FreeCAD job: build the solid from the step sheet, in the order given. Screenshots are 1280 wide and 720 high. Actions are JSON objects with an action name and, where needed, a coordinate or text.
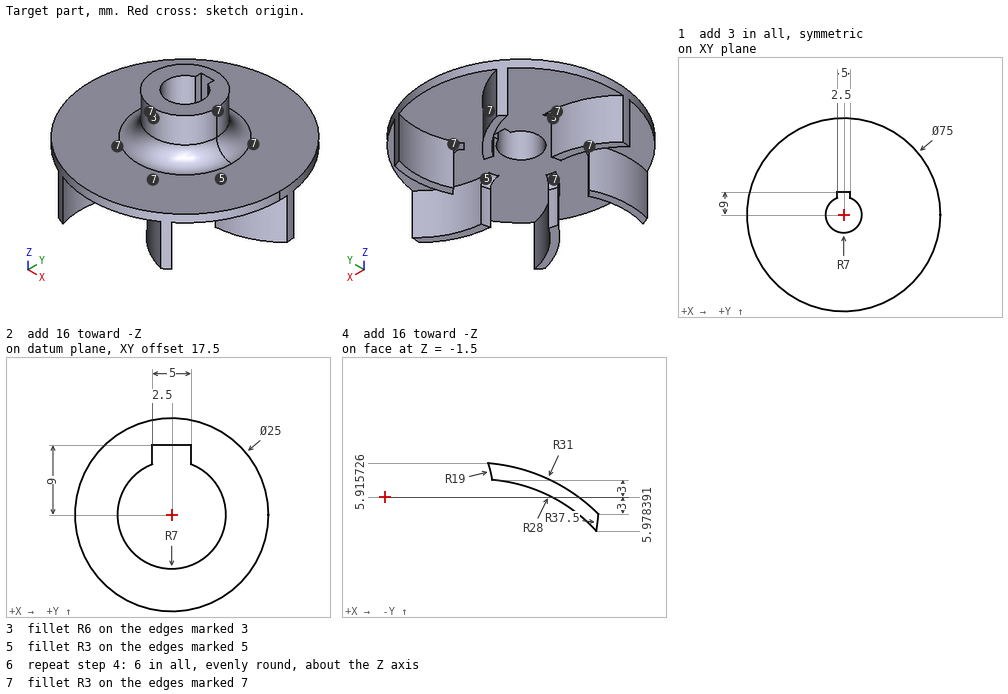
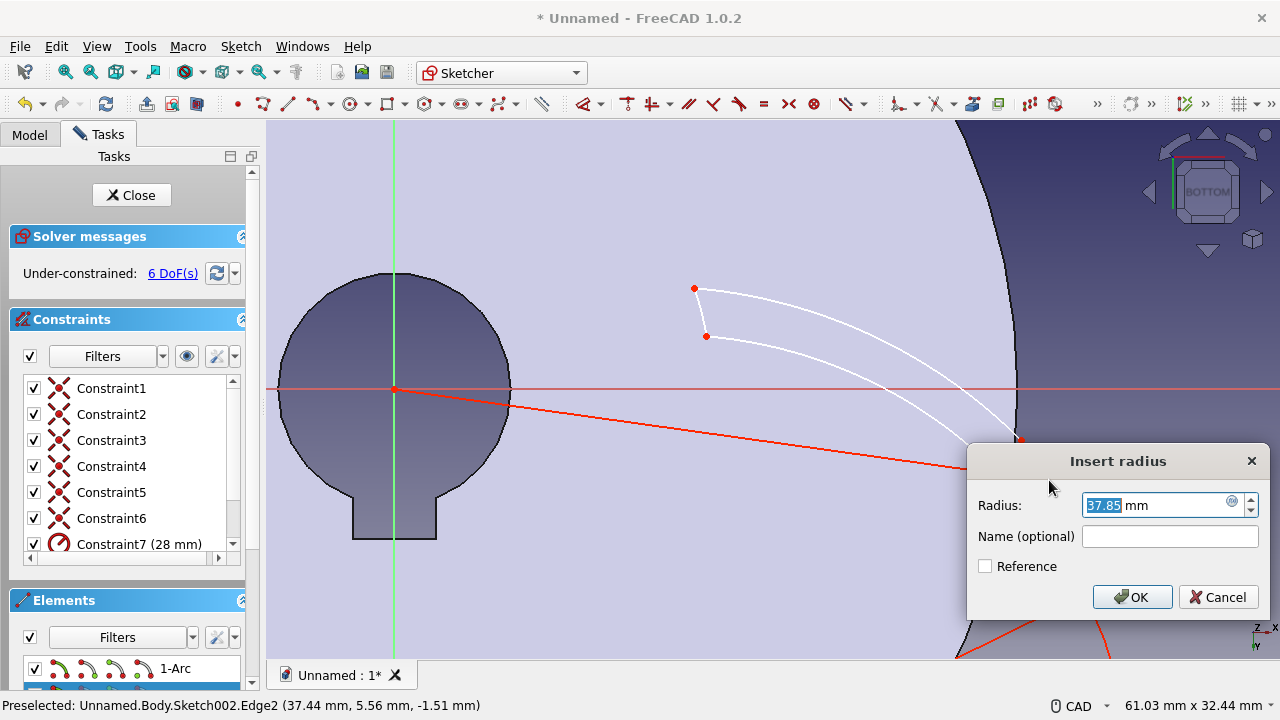
{"action": "type", "text": "37.5"}
{"action": "key", "text": "Return"}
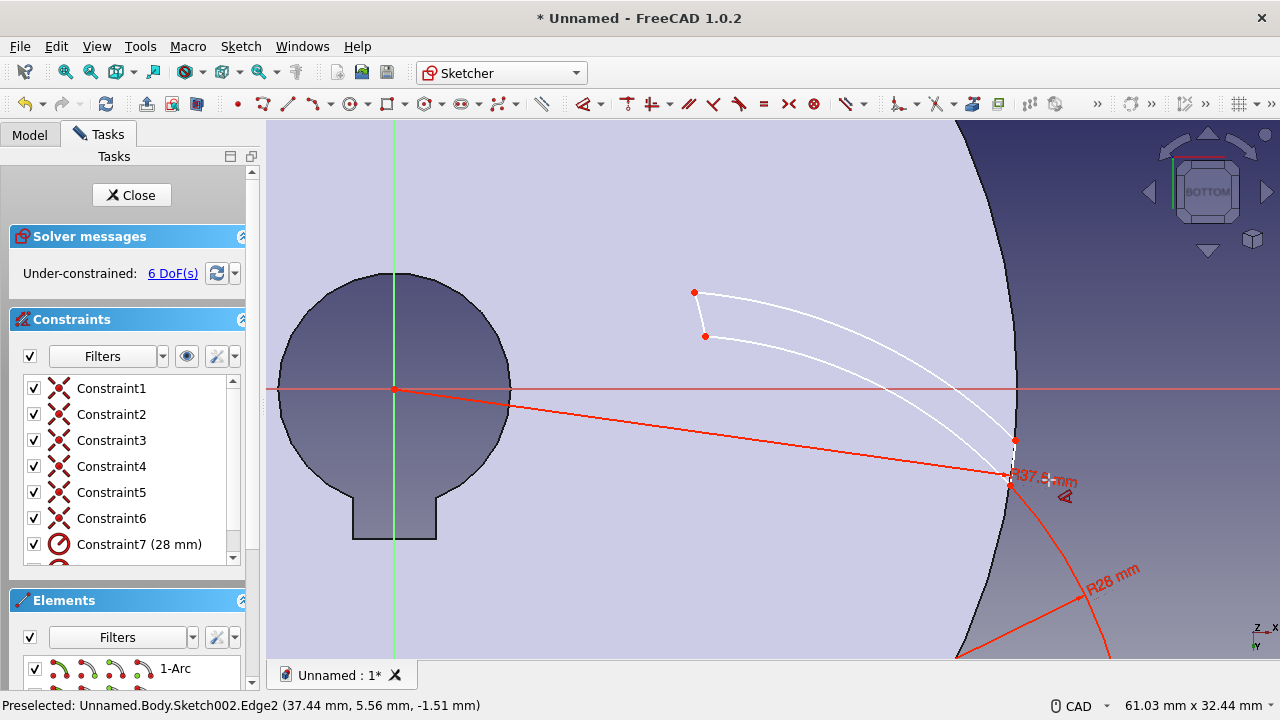
{"action": "left_click", "coordinate": [931, 373]}
{"action": "left_click", "coordinate": [948, 346]}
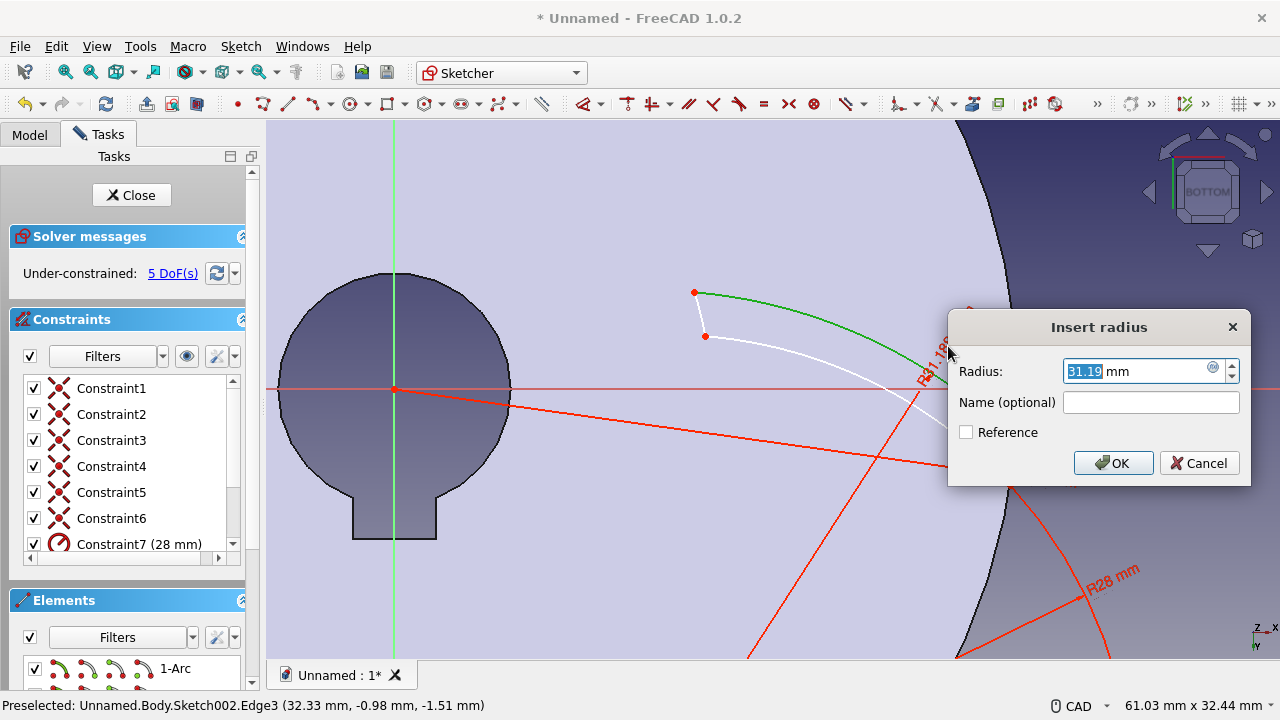
{"action": "type", "text": "31"}
{"action": "key", "text": "Return"}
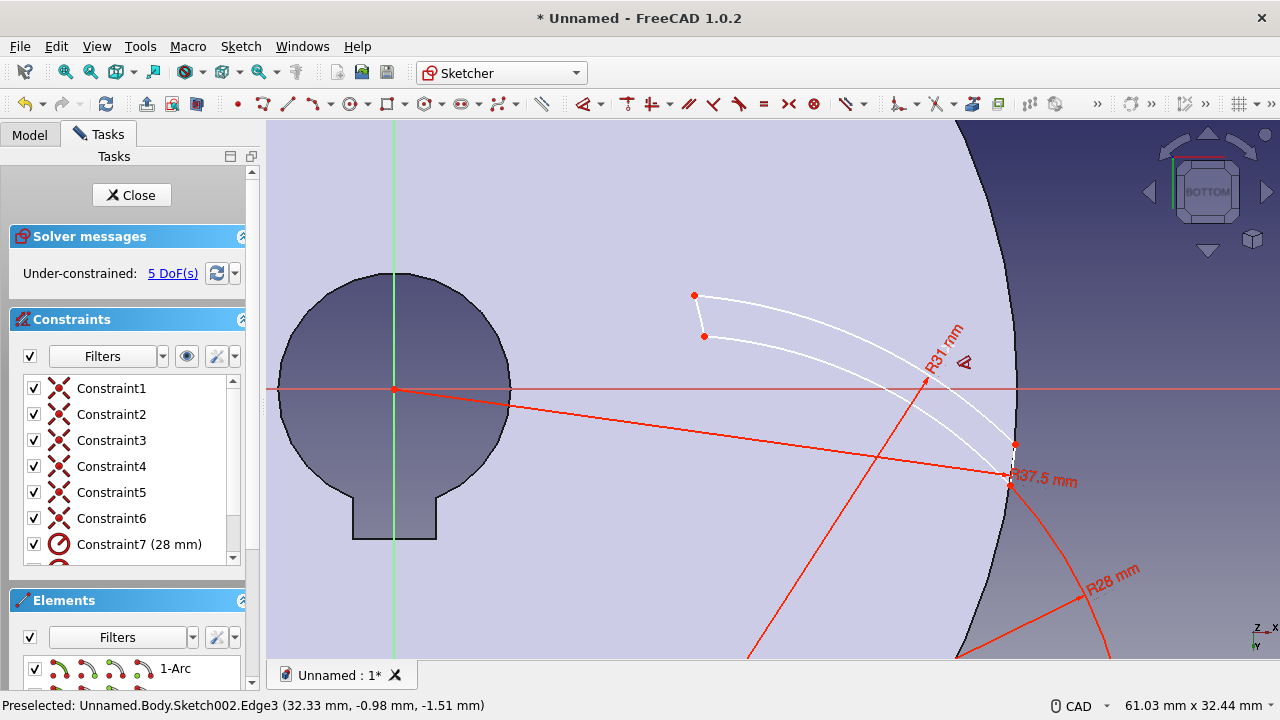
{"action": "left_click", "coordinate": [702, 324]}
{"action": "left_click", "coordinate": [733, 317]}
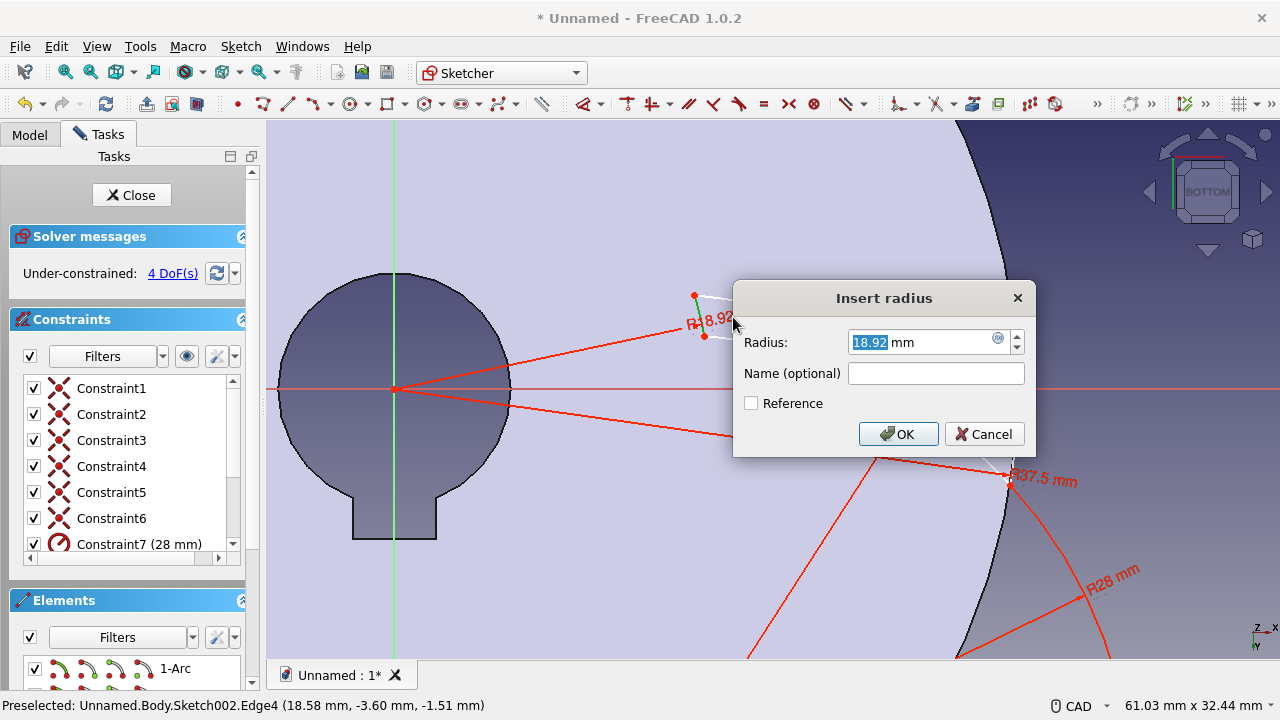
{"action": "type", "text": "19"}
{"action": "key", "text": "Return"}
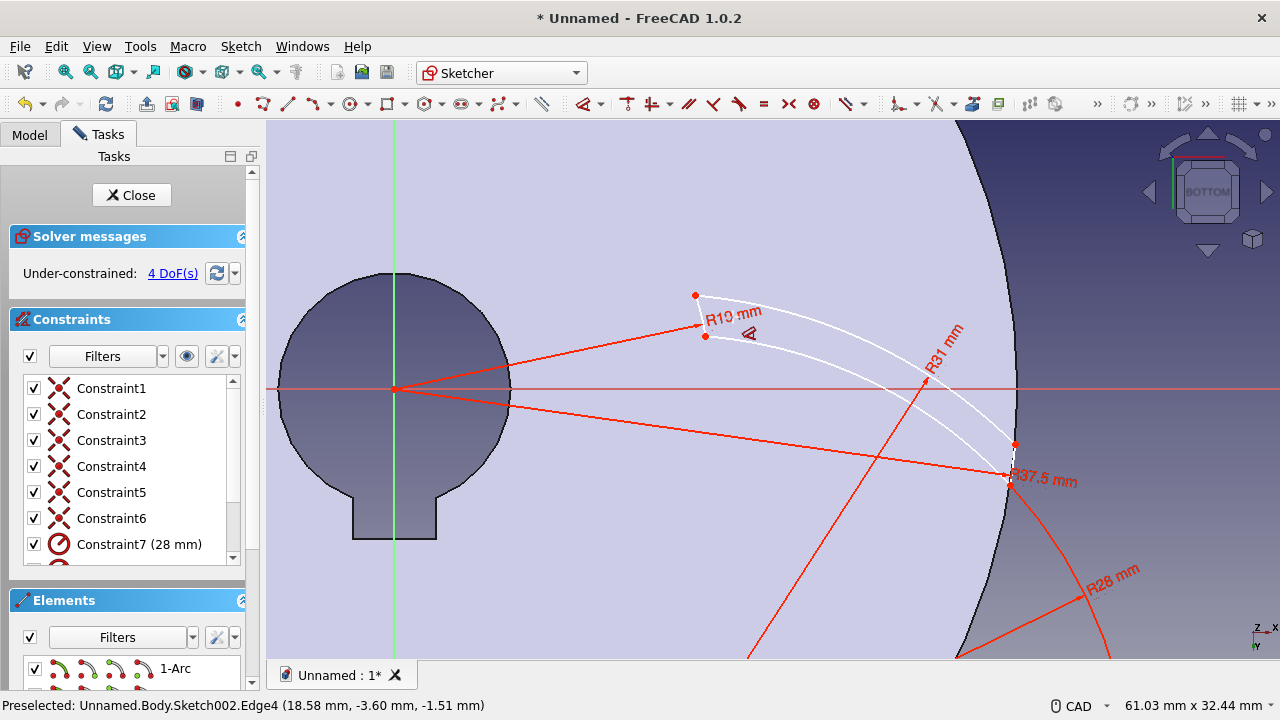
{"action": "left_click", "coordinate": [706, 336]}
{"action": "left_click", "coordinate": [360, 363]}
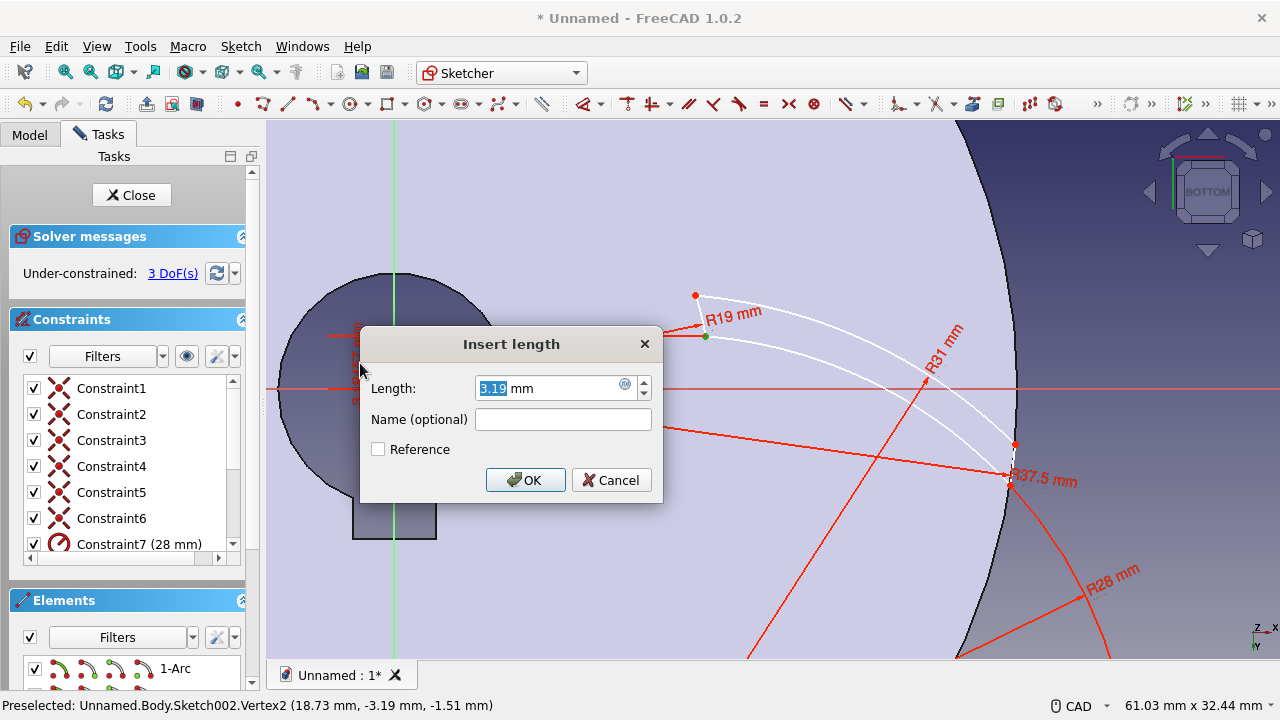
{"action": "type", "text": "3"}
{"action": "key", "text": "Return"}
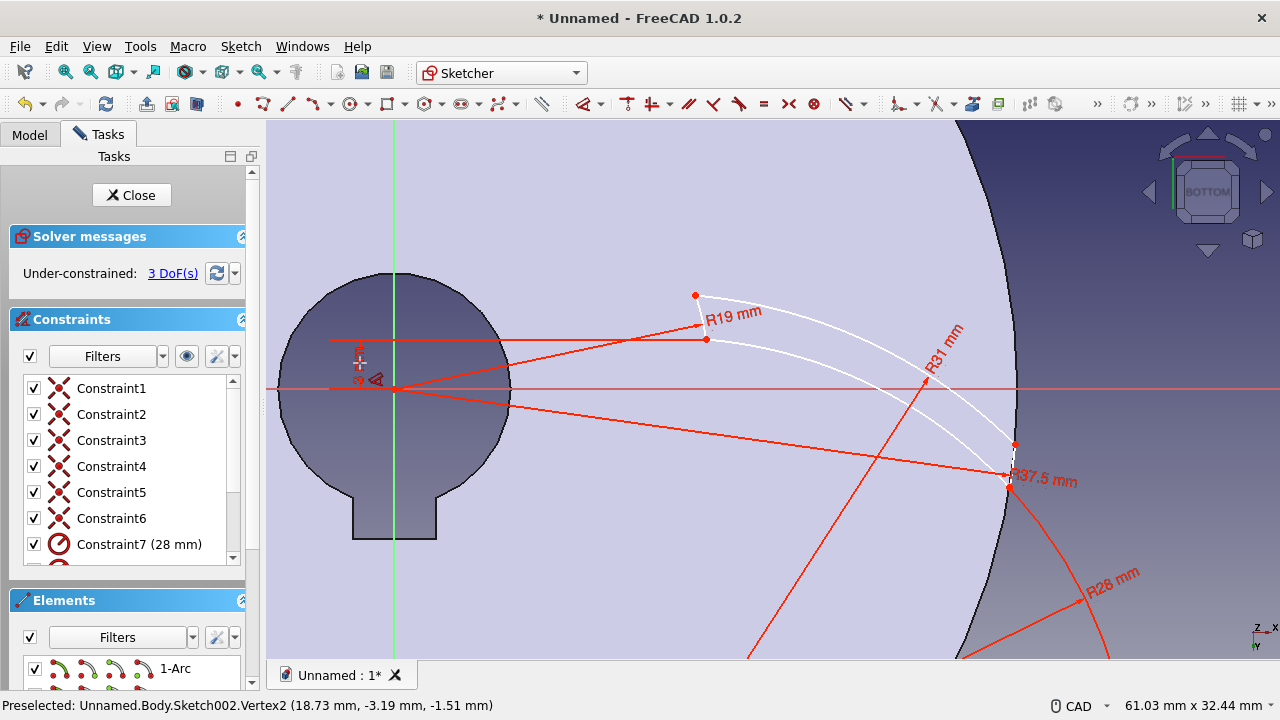
{"action": "left_click", "coordinate": [1015, 445]}
{"action": "left_click", "coordinate": [360, 417]}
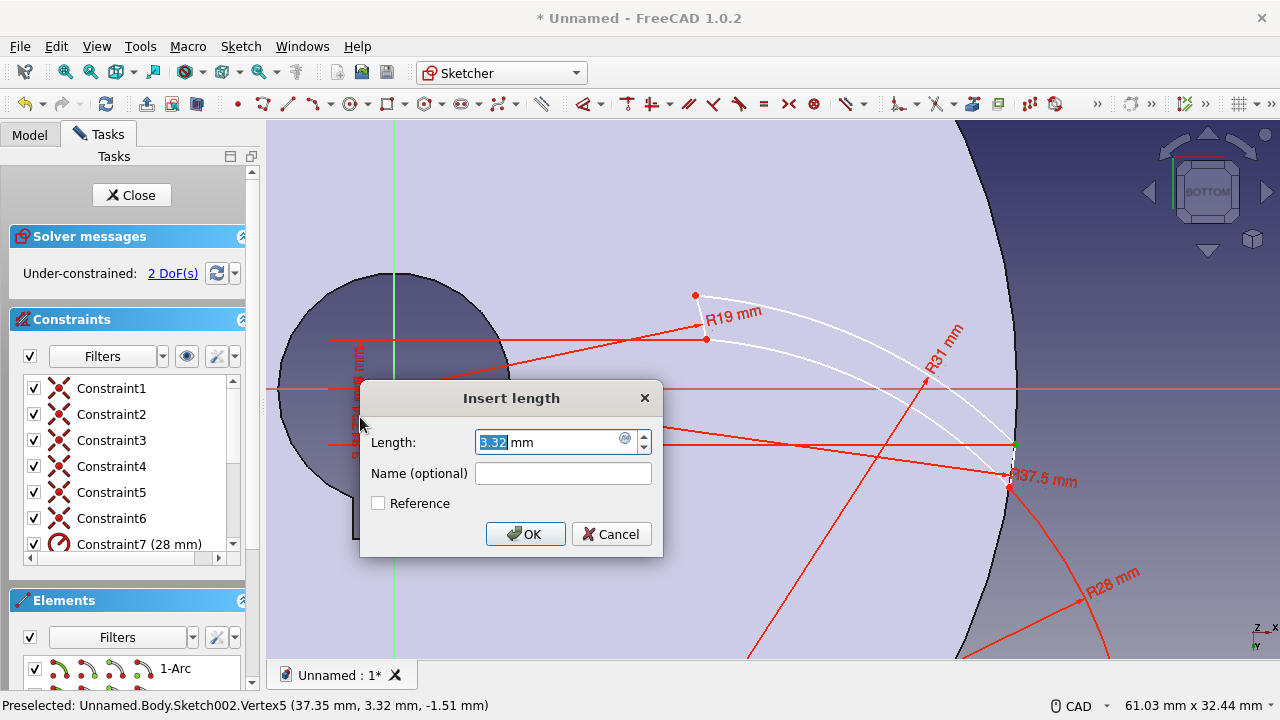
{"action": "type", "text": "3"}
{"action": "key", "text": "Return"}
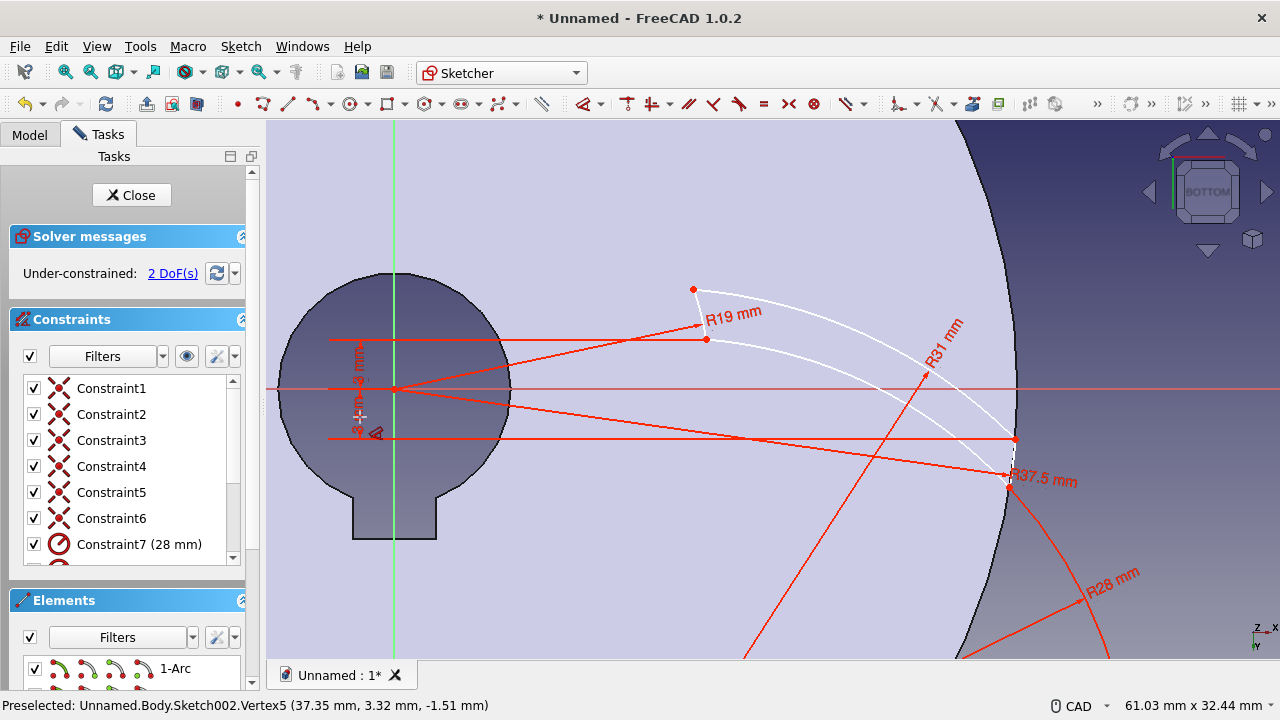
{"action": "left_click", "coordinate": [1010, 488]}
{"action": "left_click", "coordinate": [360, 439]}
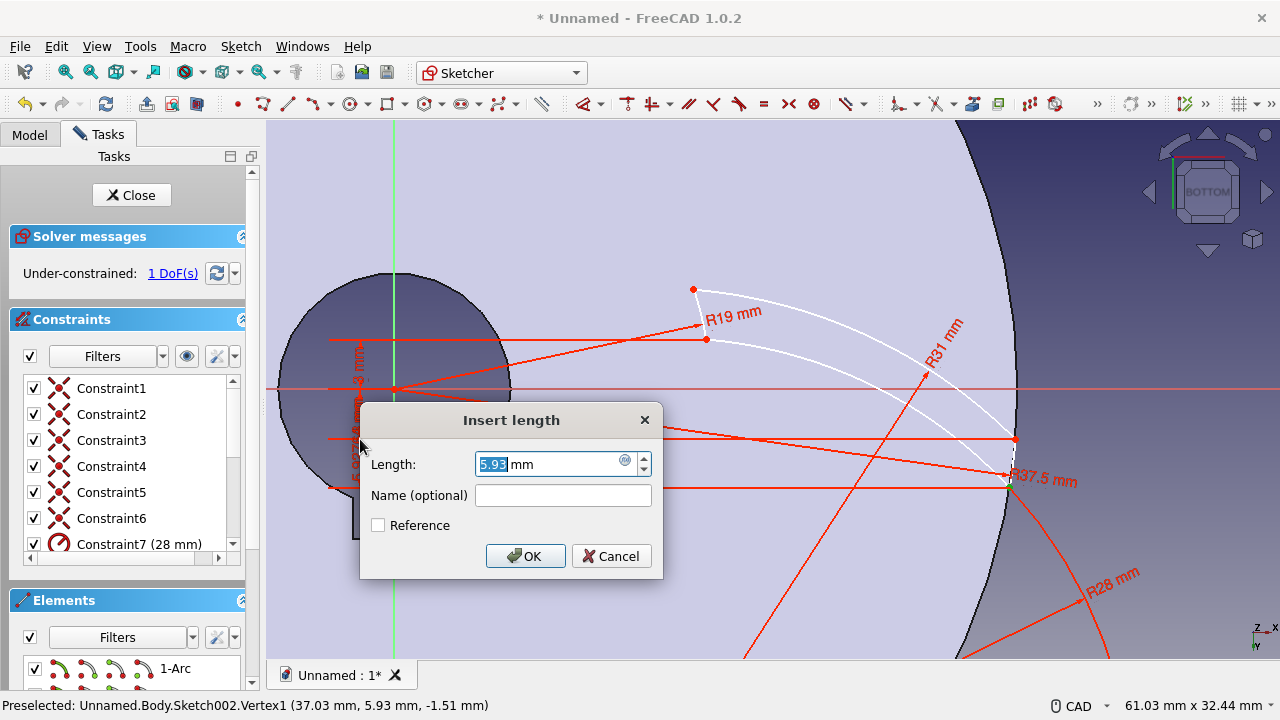
{"action": "type", "text": "5.978391"}
{"action": "key", "text": "Return"}